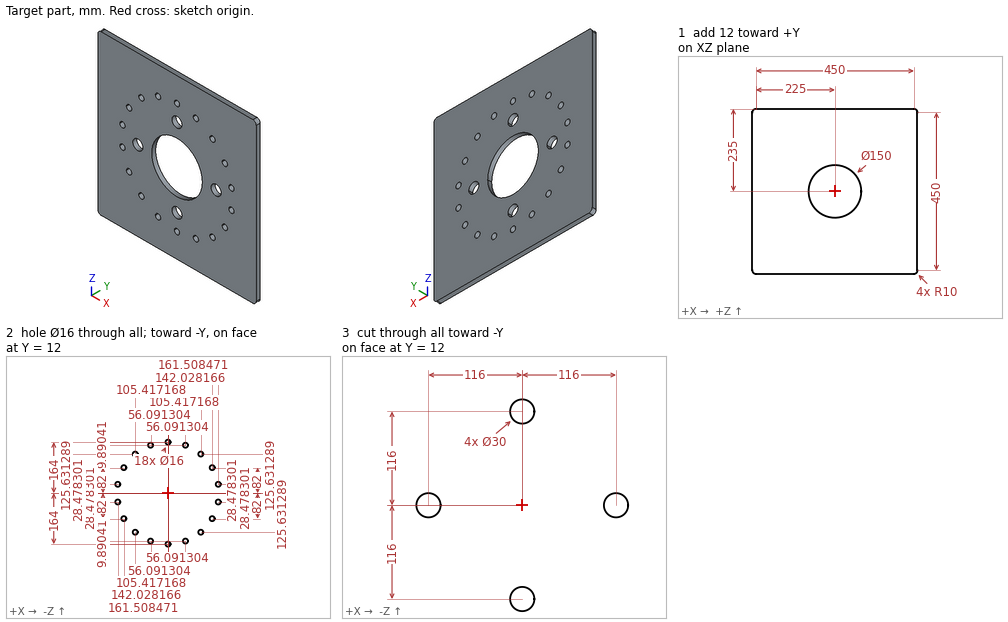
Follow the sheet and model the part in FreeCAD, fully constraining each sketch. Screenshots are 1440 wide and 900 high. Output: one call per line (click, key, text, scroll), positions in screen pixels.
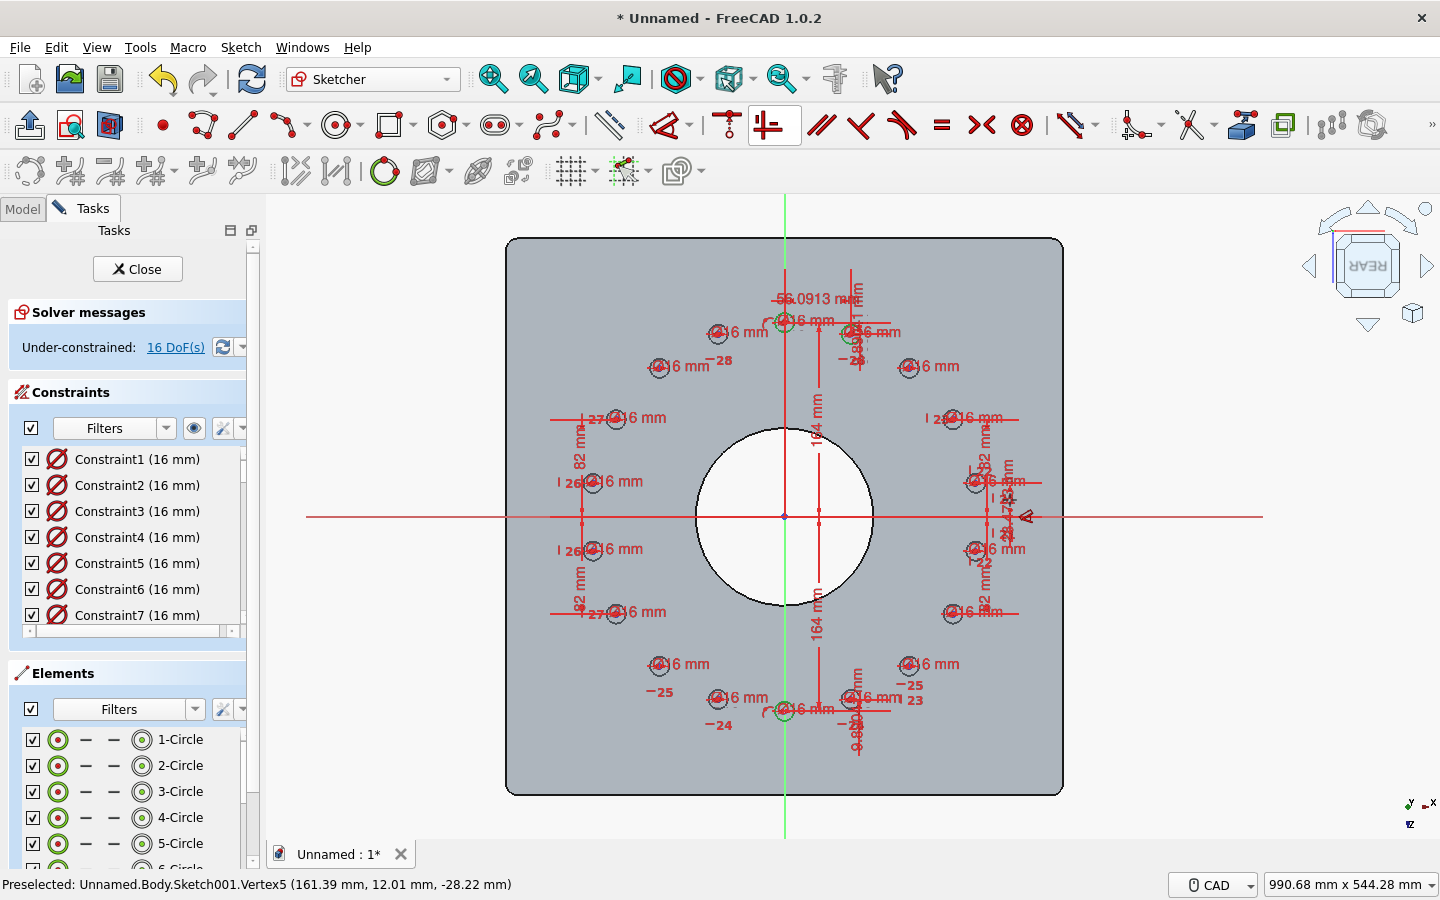
click(976, 551)
click(1010, 534)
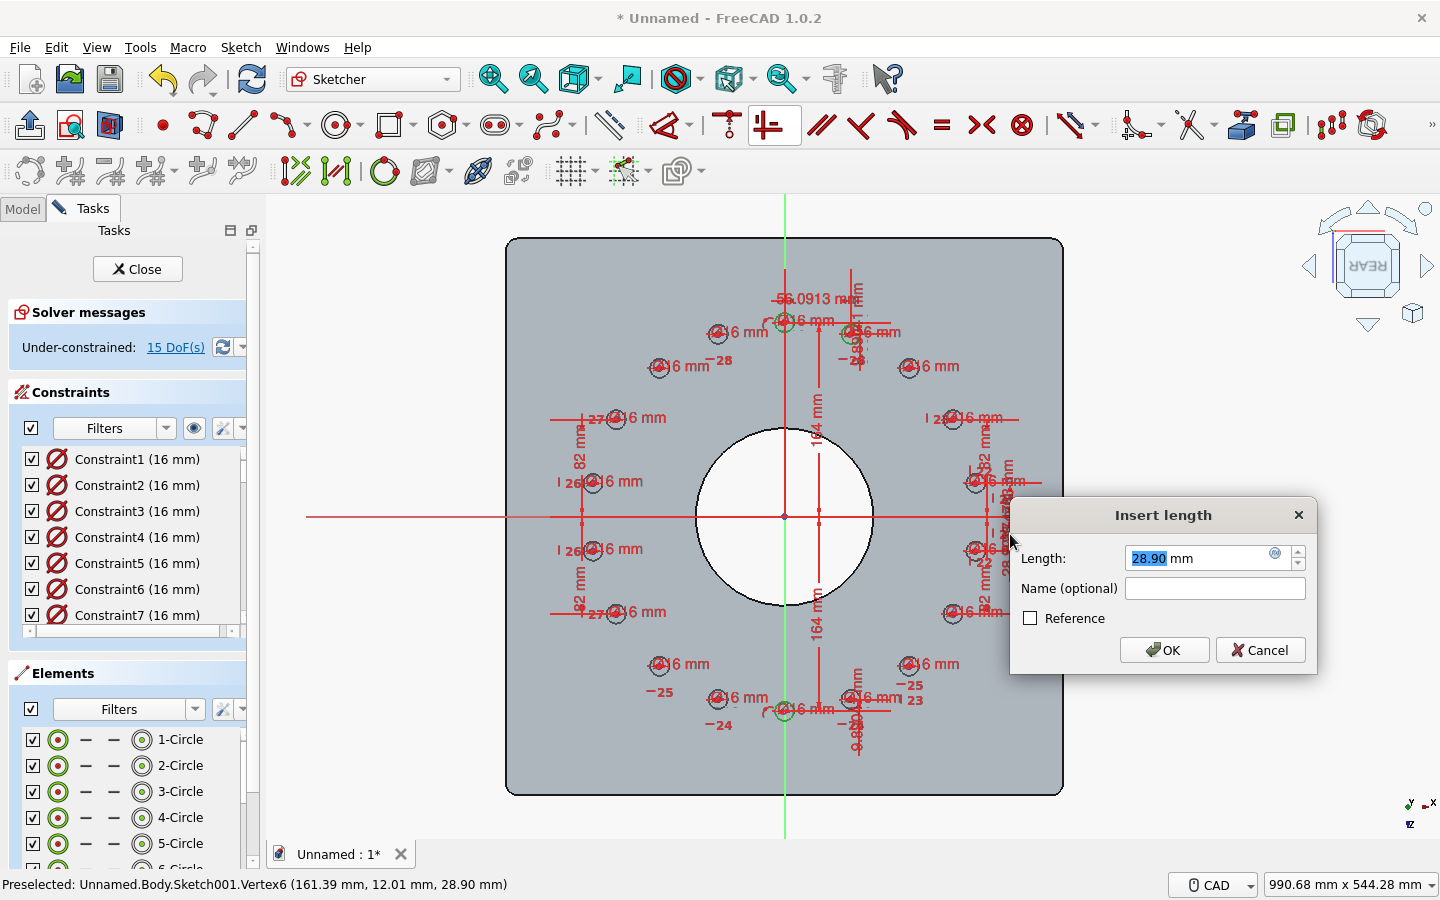
text(28.478301)
key(Return)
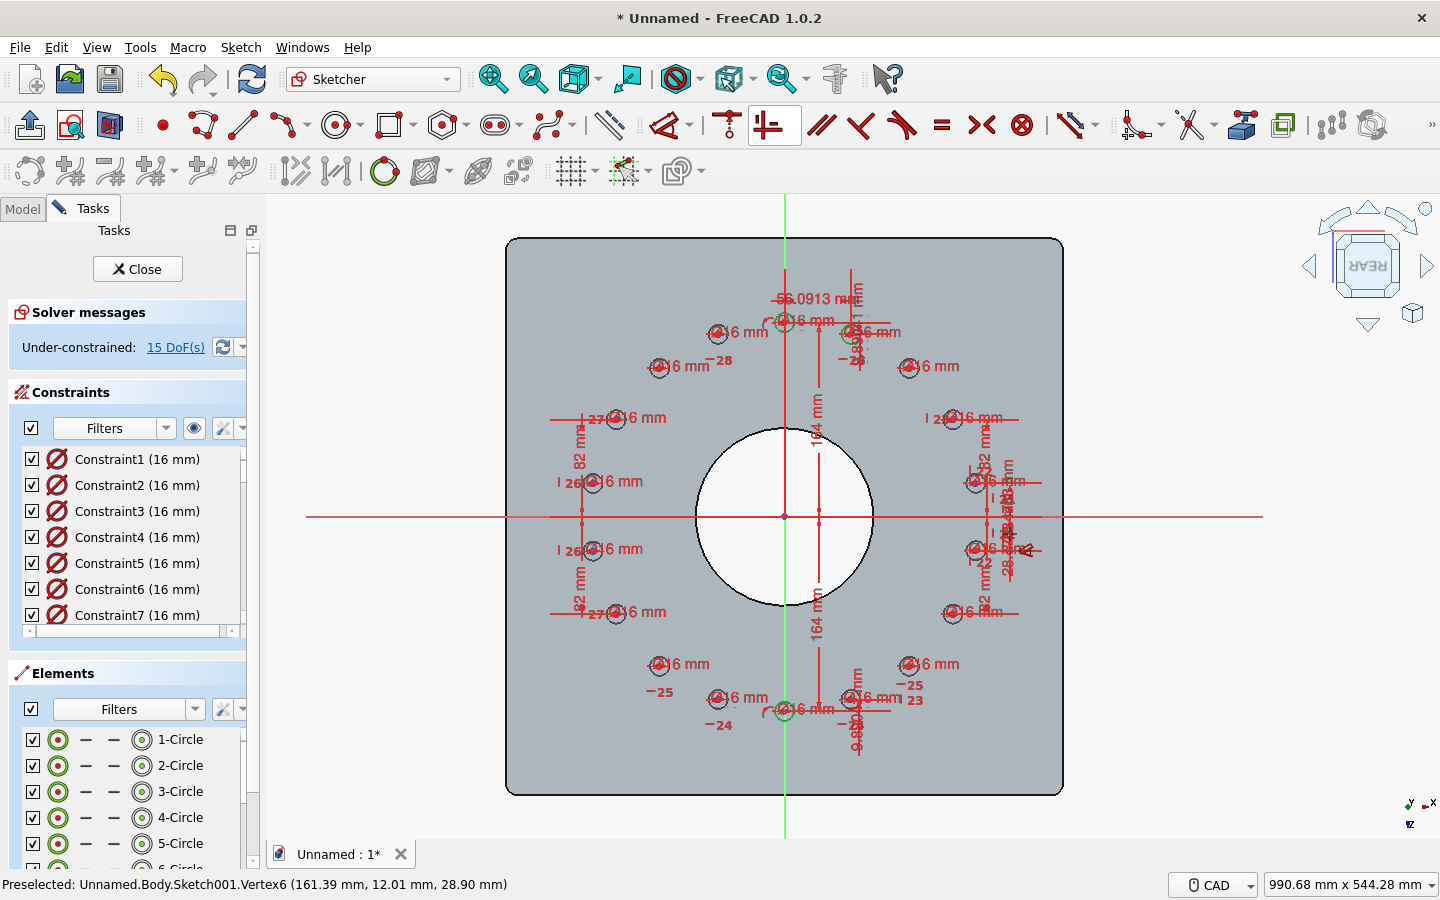
click(851, 700)
click(818, 734)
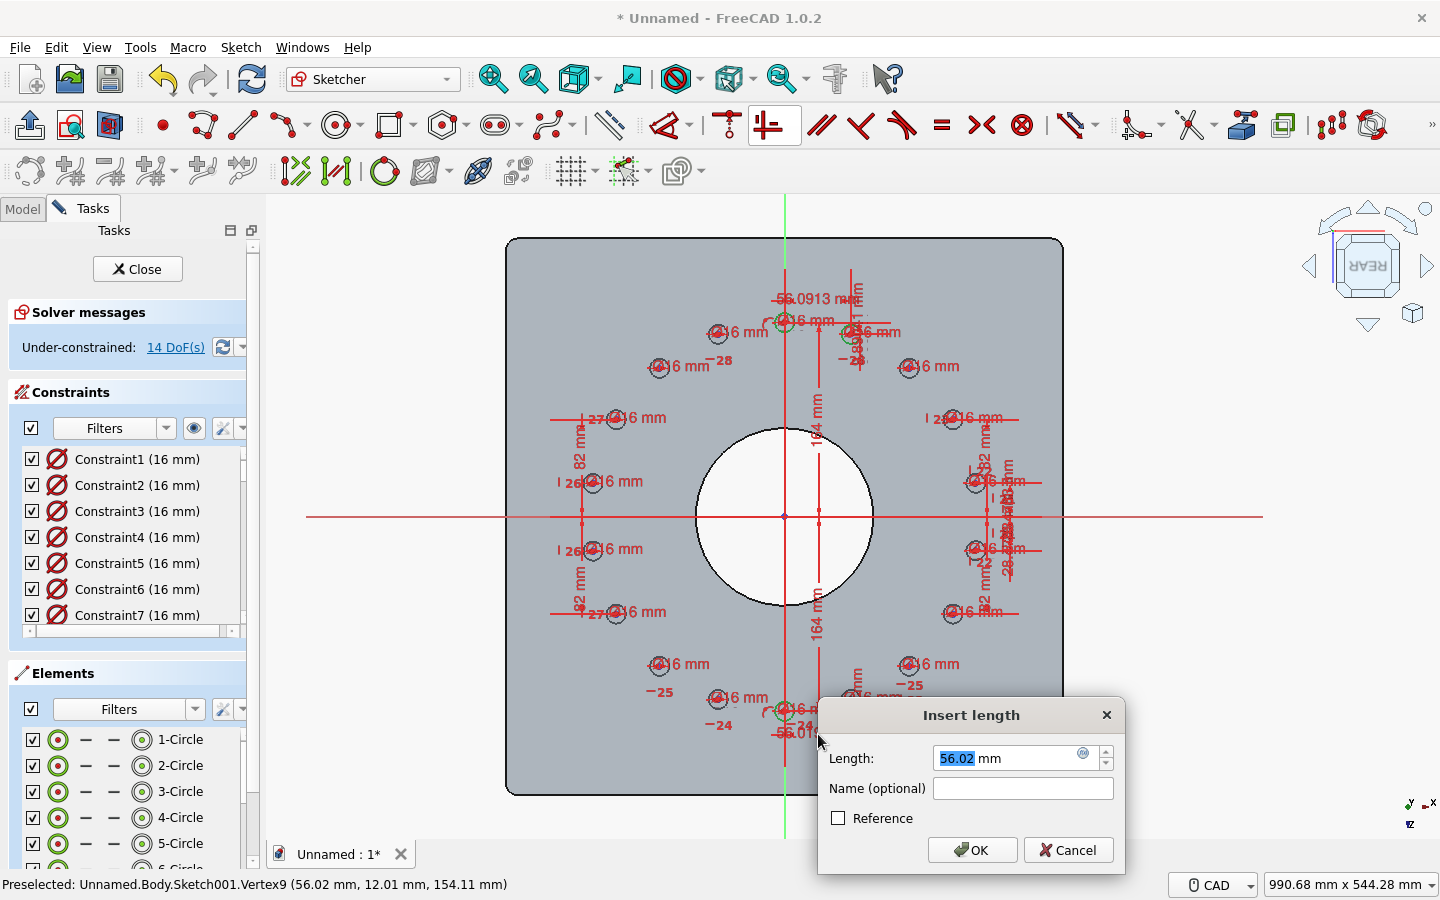
text(56.091304)
key(Return)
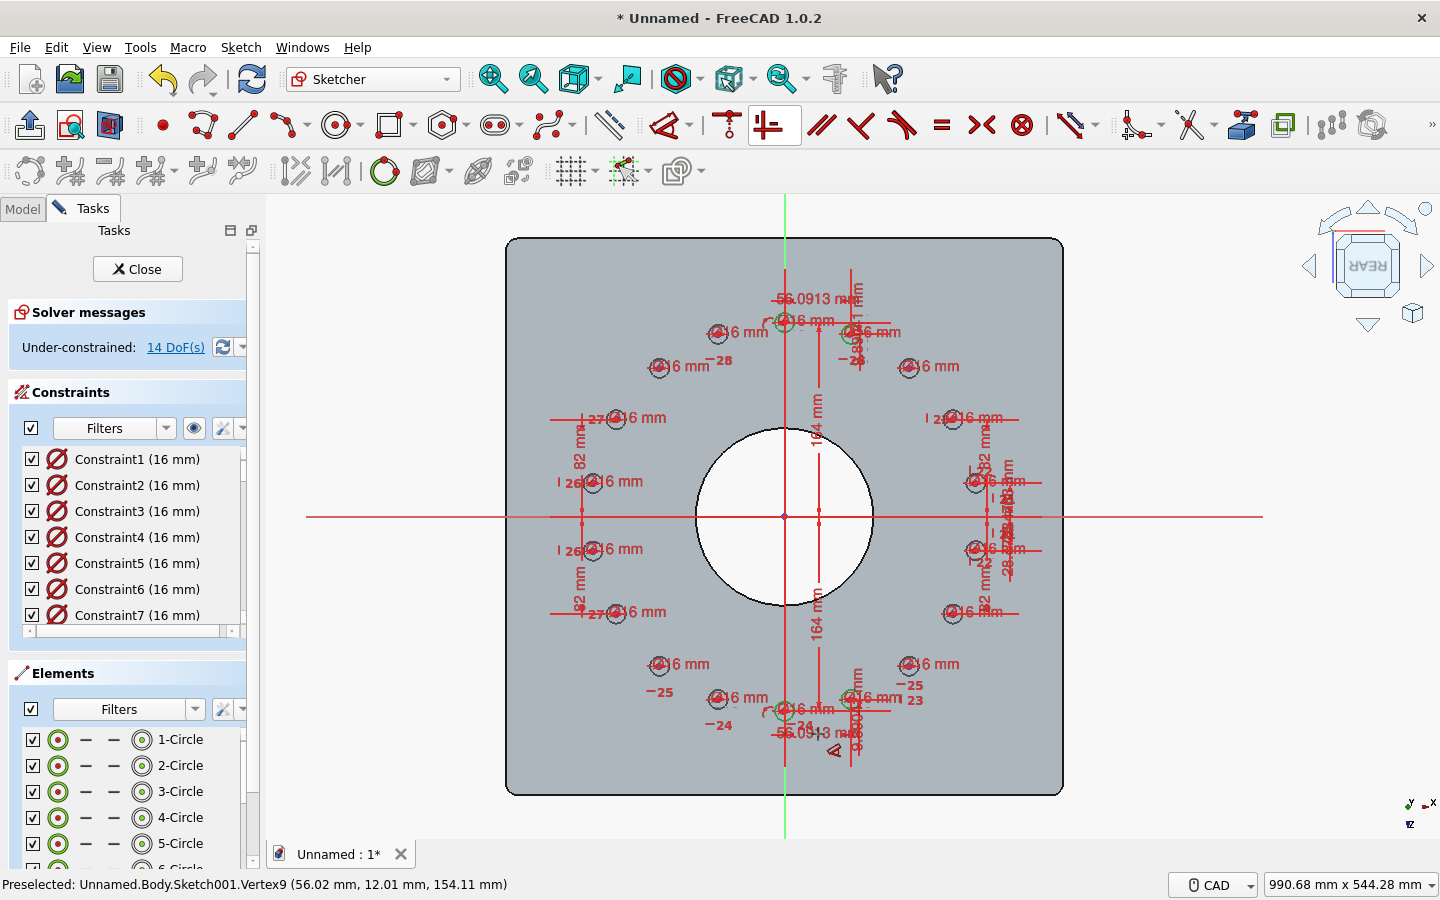
click(718, 700)
click(736, 734)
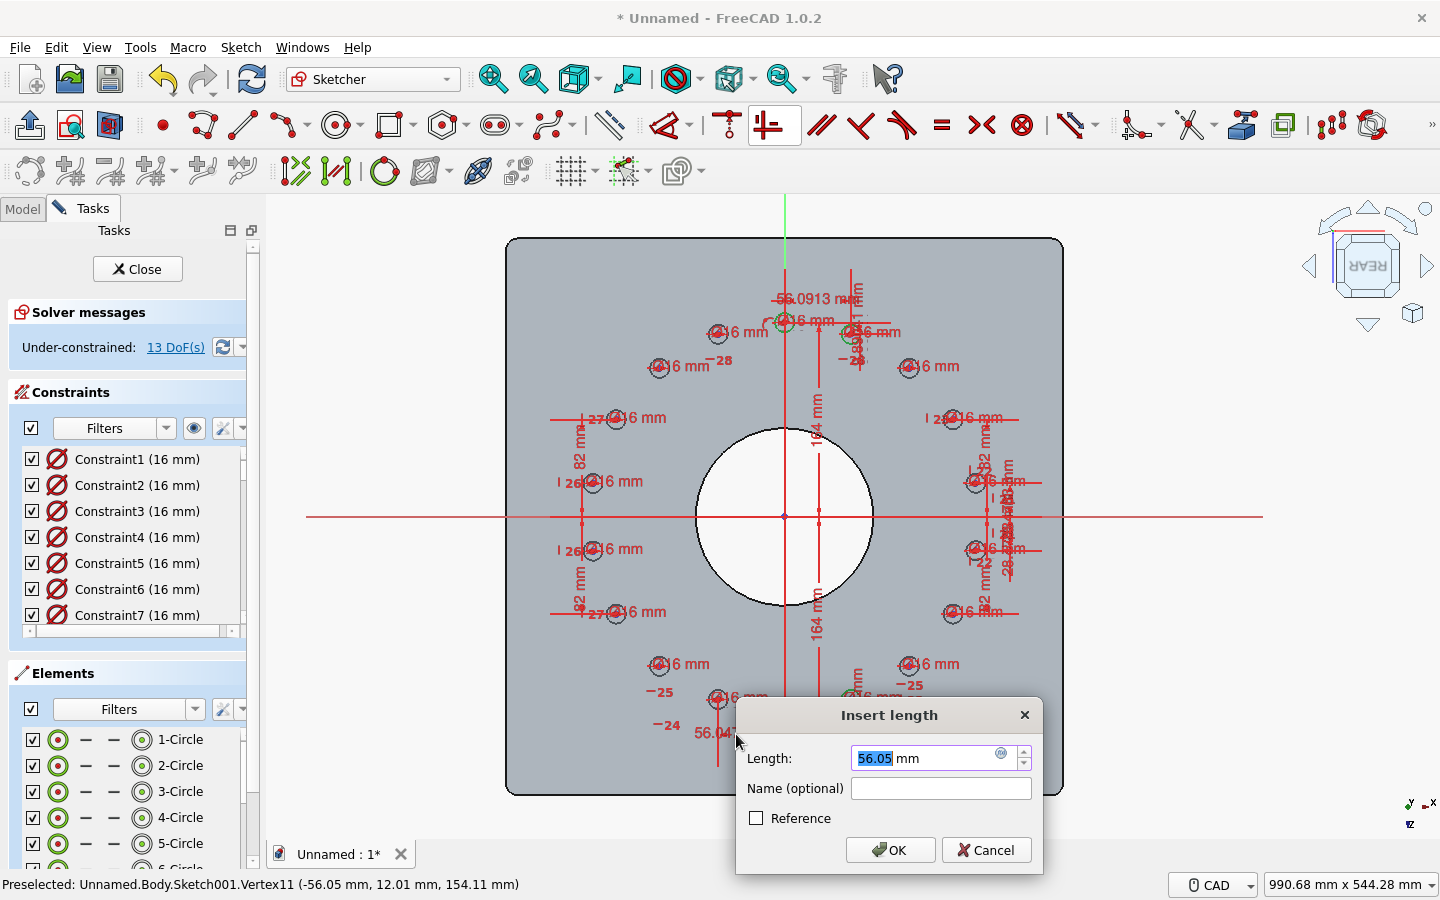
text(56.091304)
key(Return)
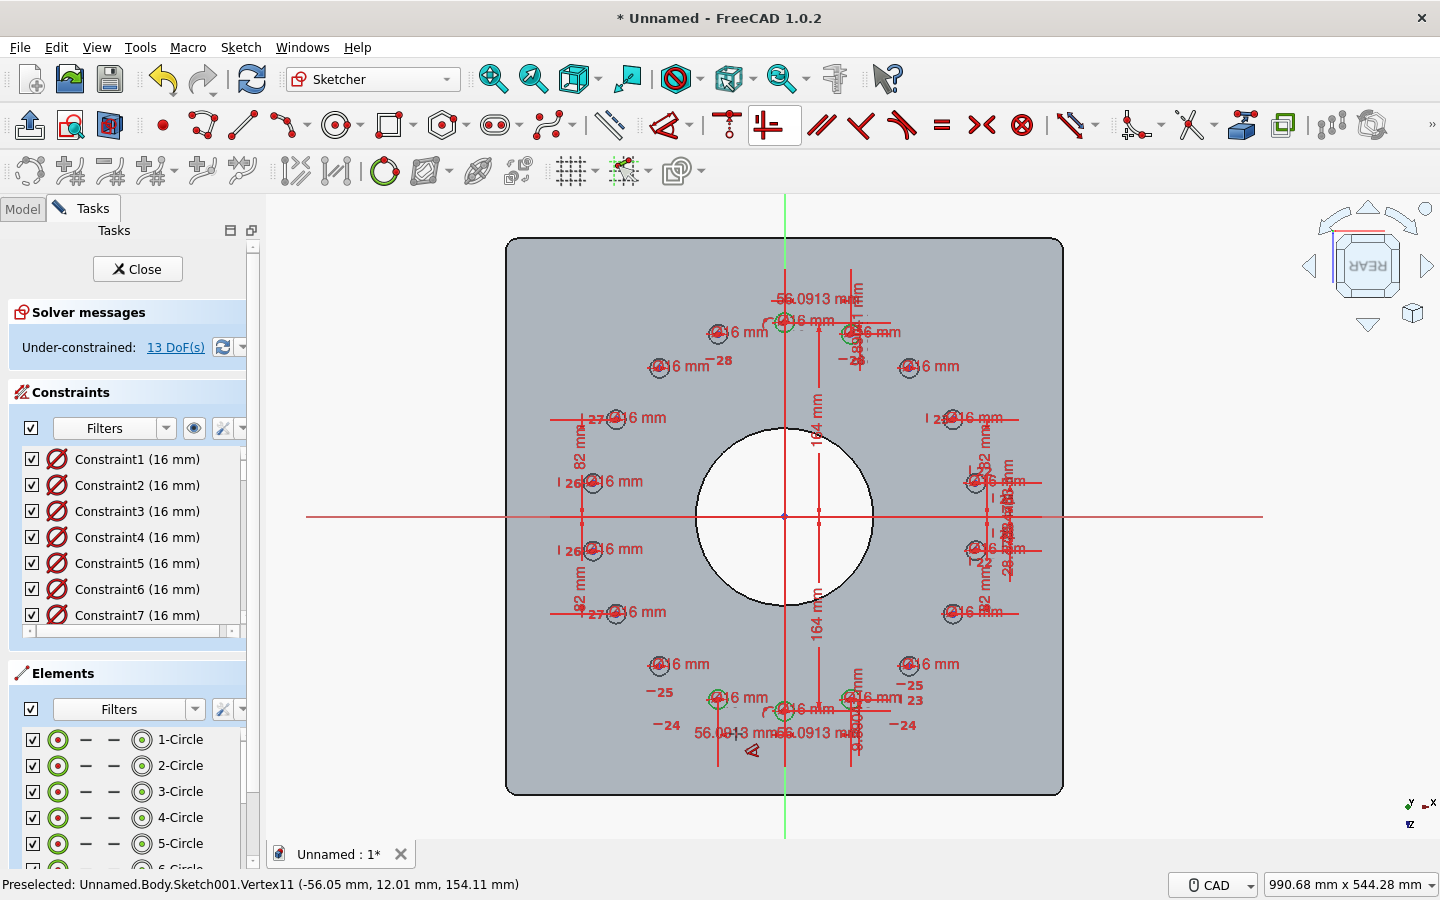
click(593, 551)
click(559, 534)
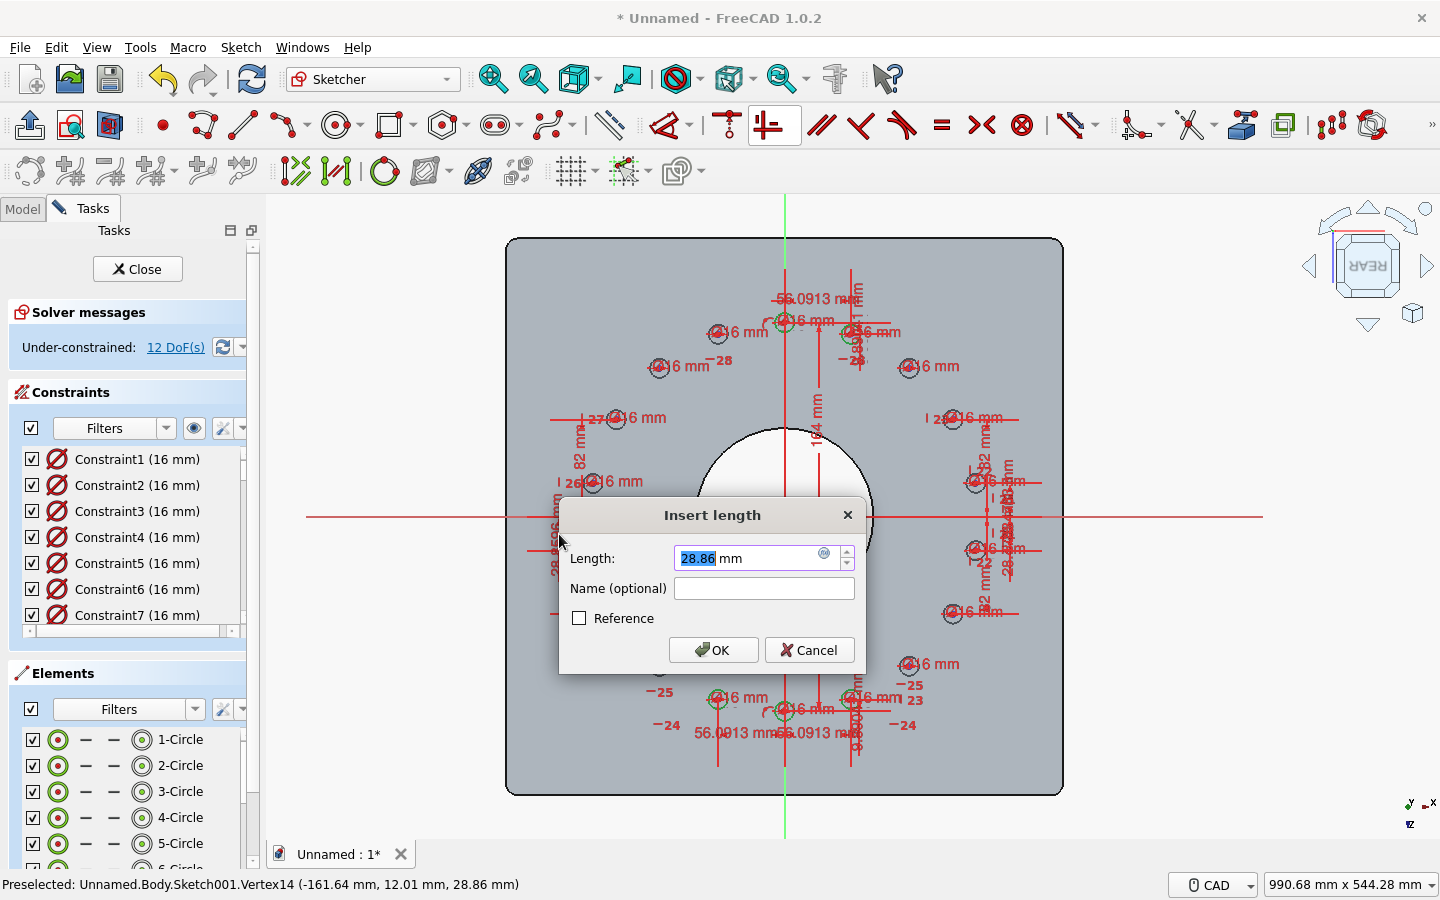
text(28.478301)
key(Return)